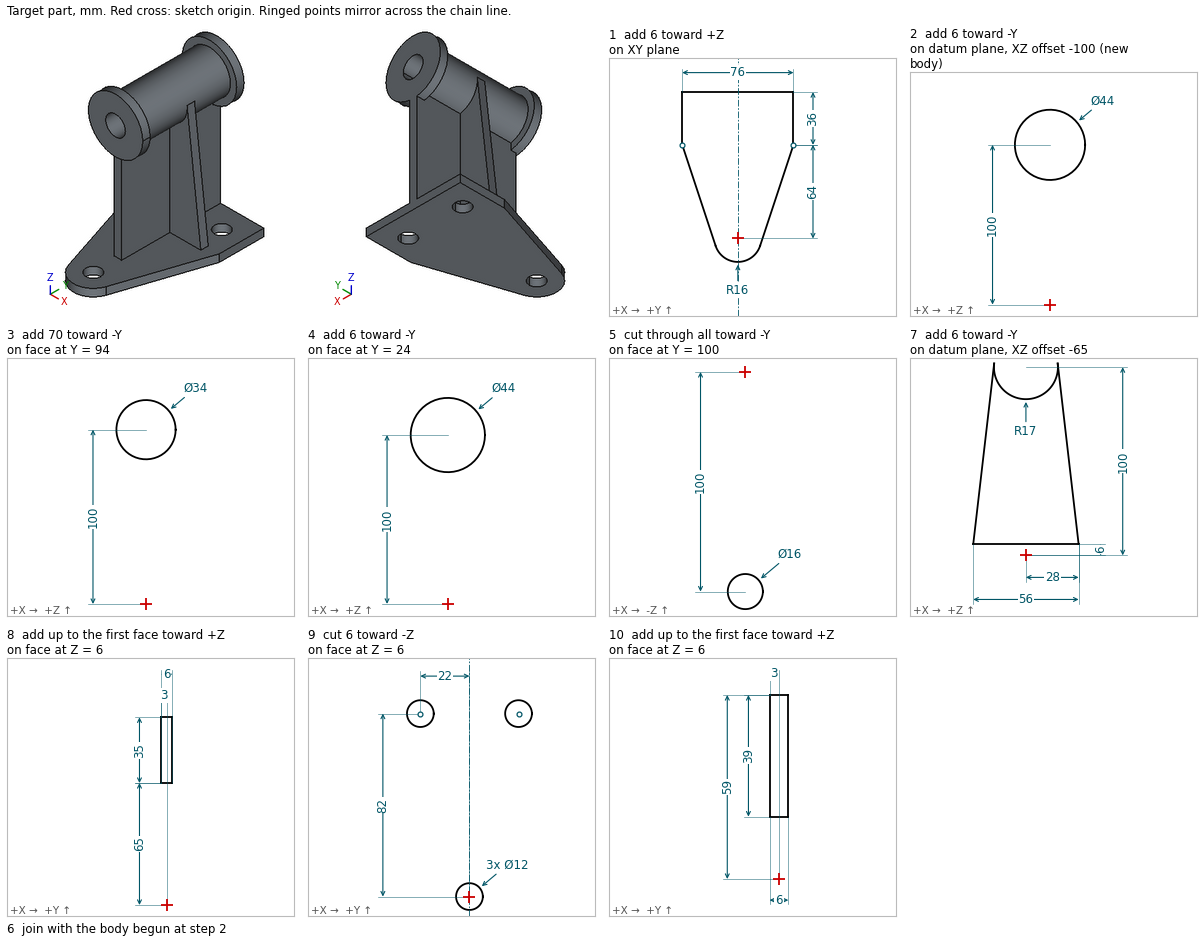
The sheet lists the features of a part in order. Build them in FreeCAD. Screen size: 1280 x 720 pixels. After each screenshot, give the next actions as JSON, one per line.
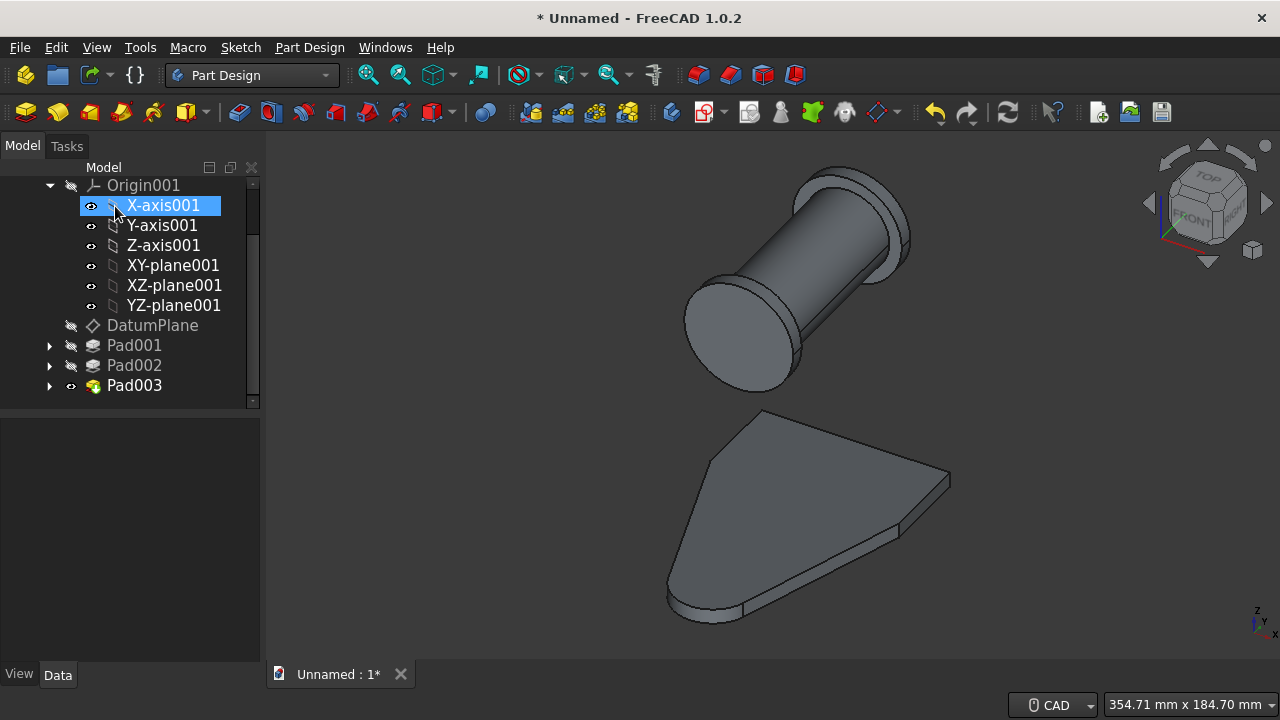
{"action": "key", "text": "4"}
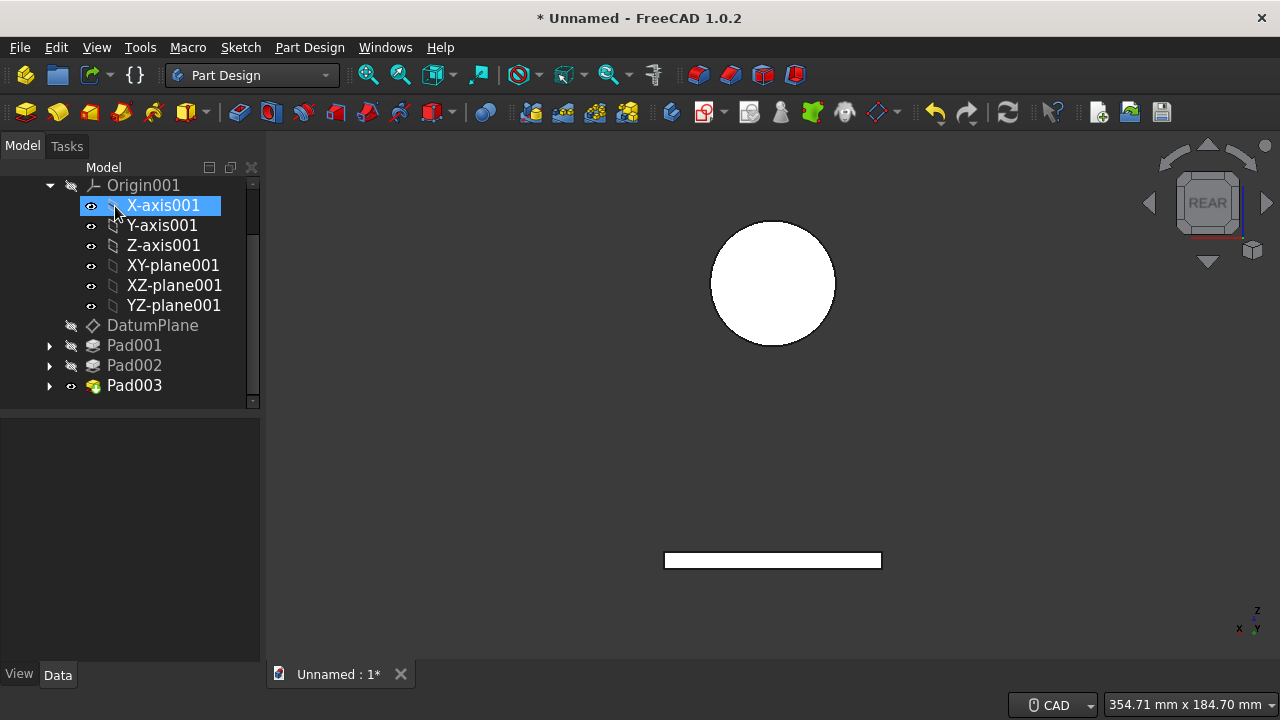
{"action": "left_click", "coordinate": [370, 76]}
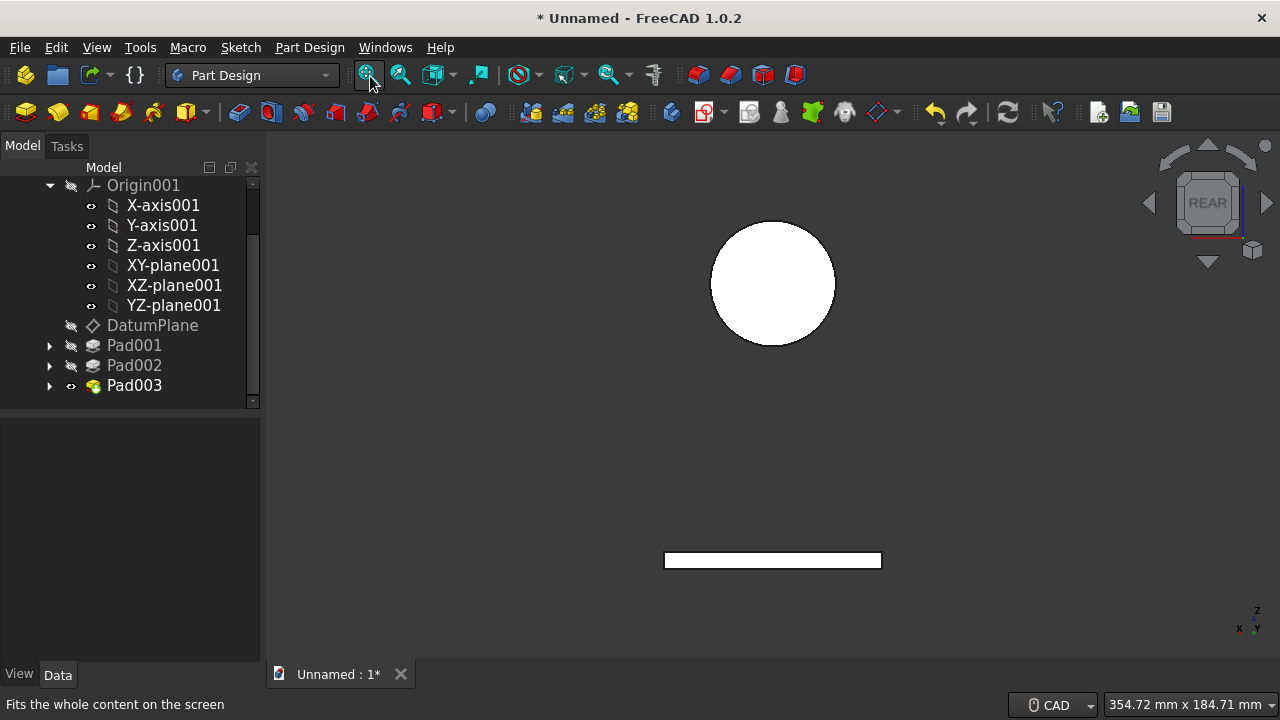
{"action": "left_click", "coordinate": [773, 283]}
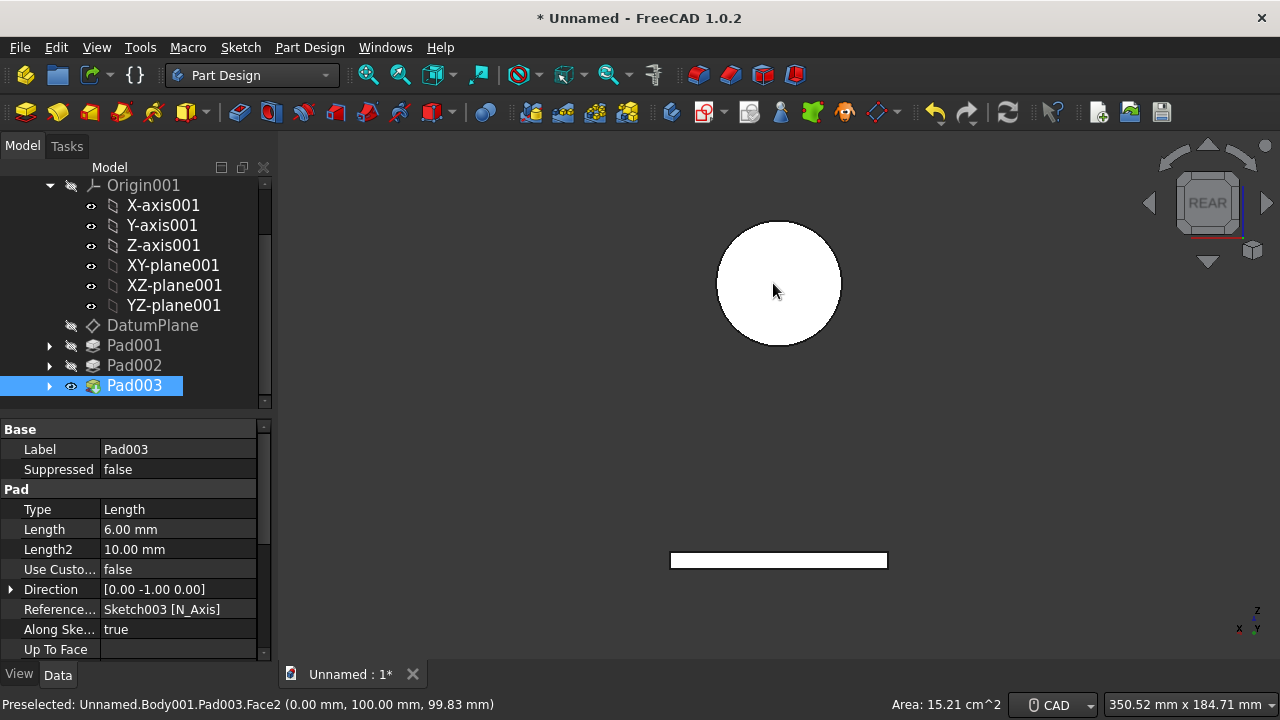
{"action": "left_click", "coordinate": [704, 112]}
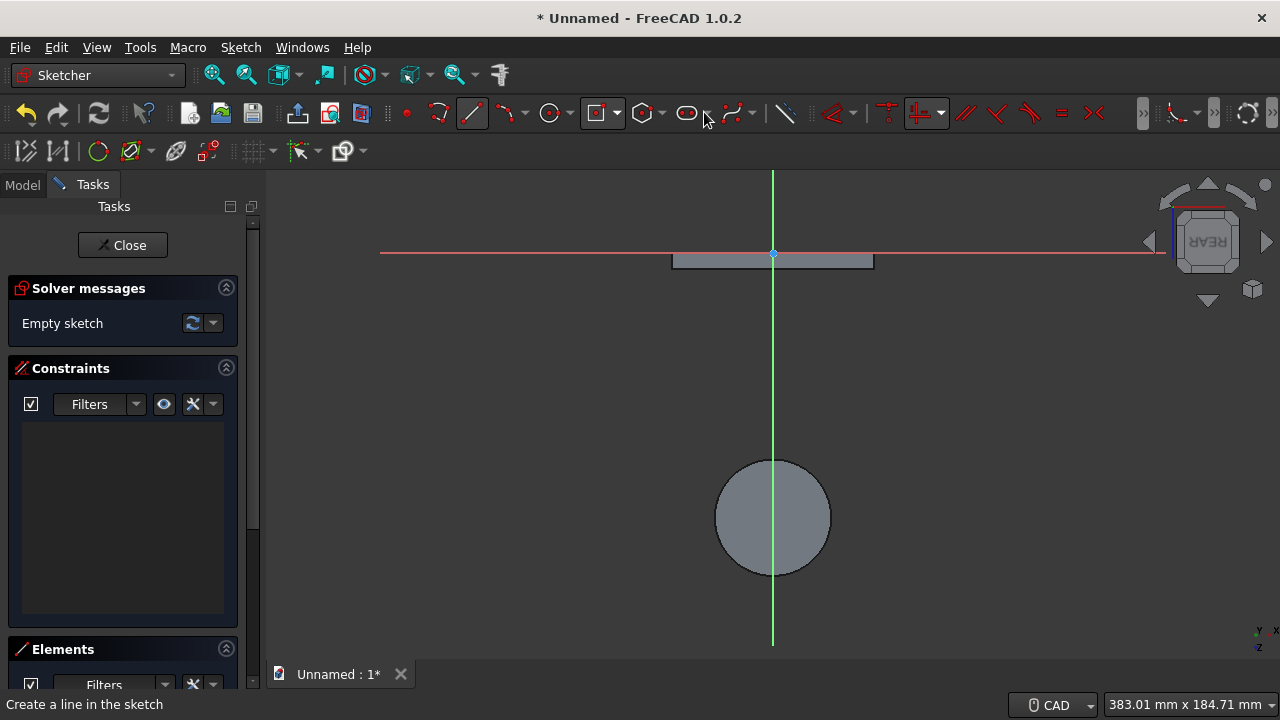
{"action": "scroll", "coordinate": [784, 534], "scroll_direction": "up", "scroll_amount": 10}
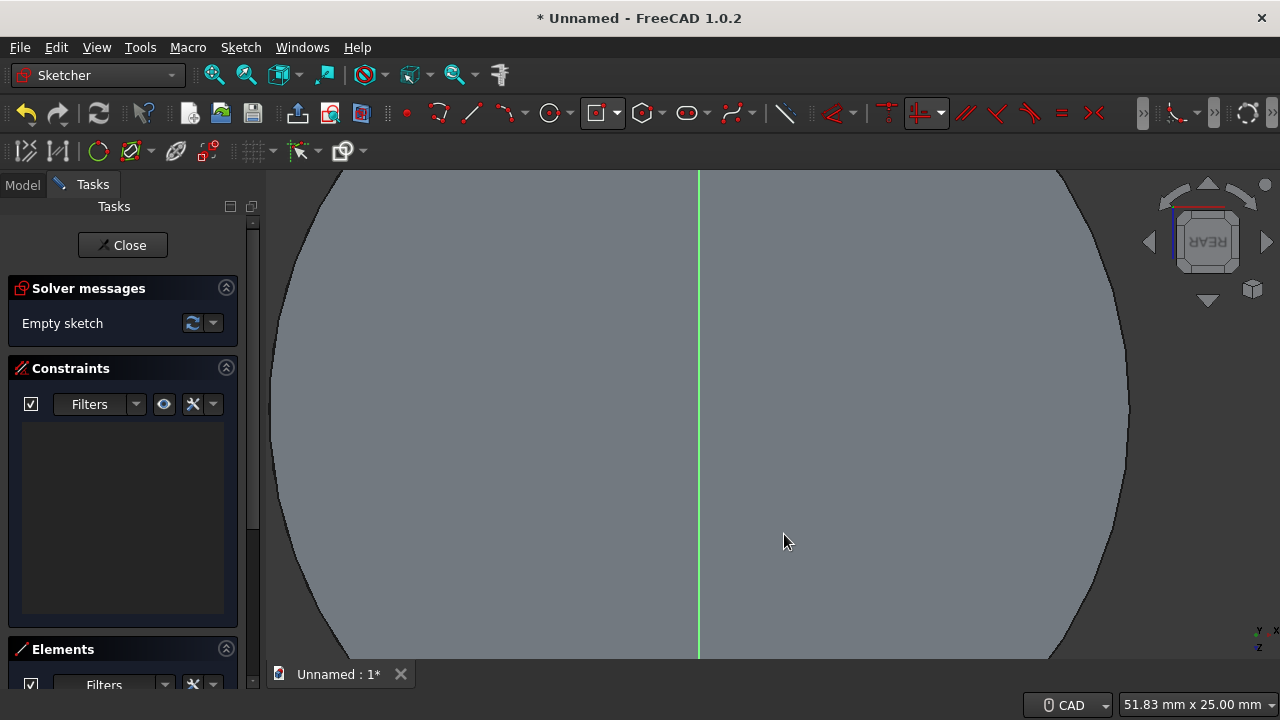
{"action": "key", "text": "g c"}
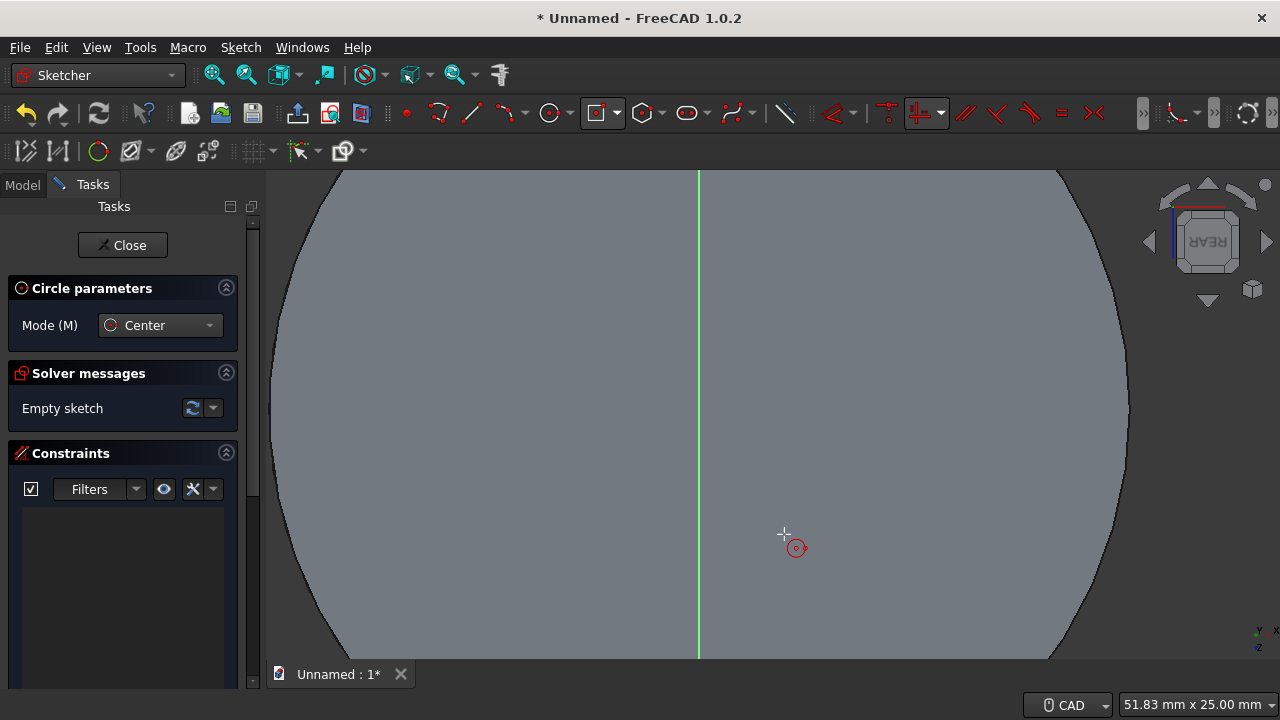
{"action": "left_click", "coordinate": [699, 409]}
{"action": "left_click", "coordinate": [810, 299]}
{"action": "key", "text": "Escape"}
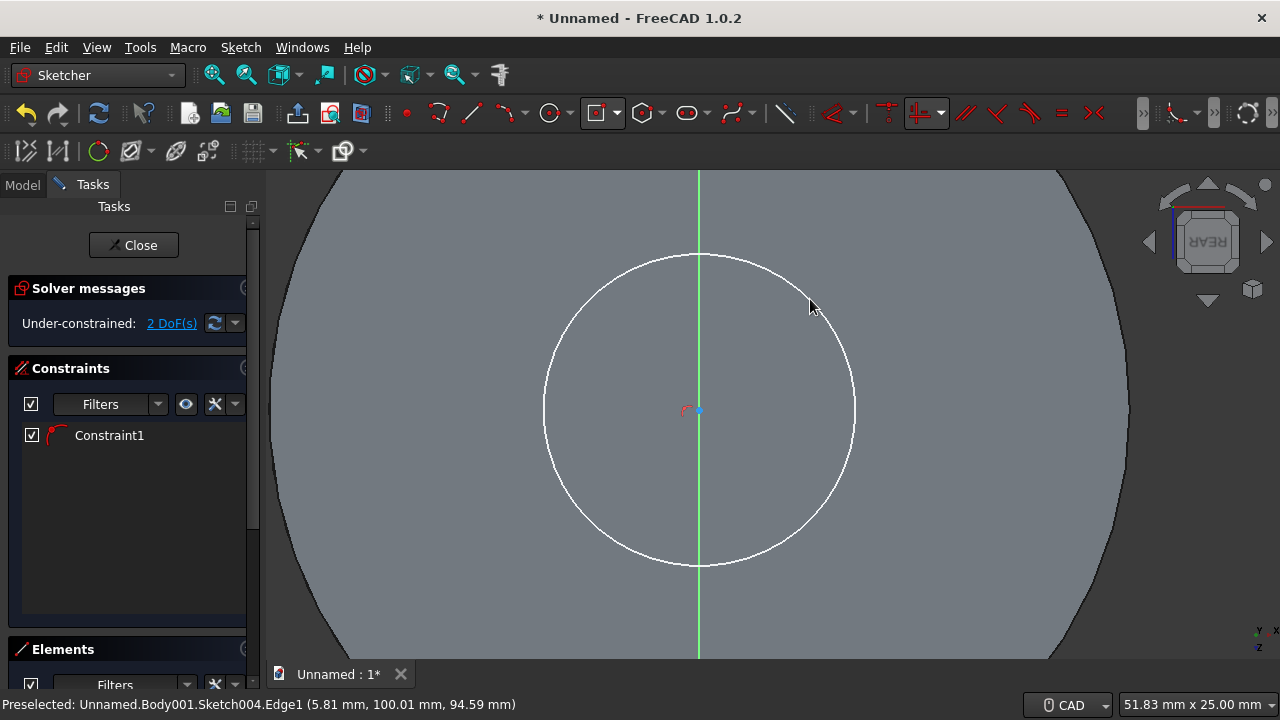
{"action": "key", "text": "d"}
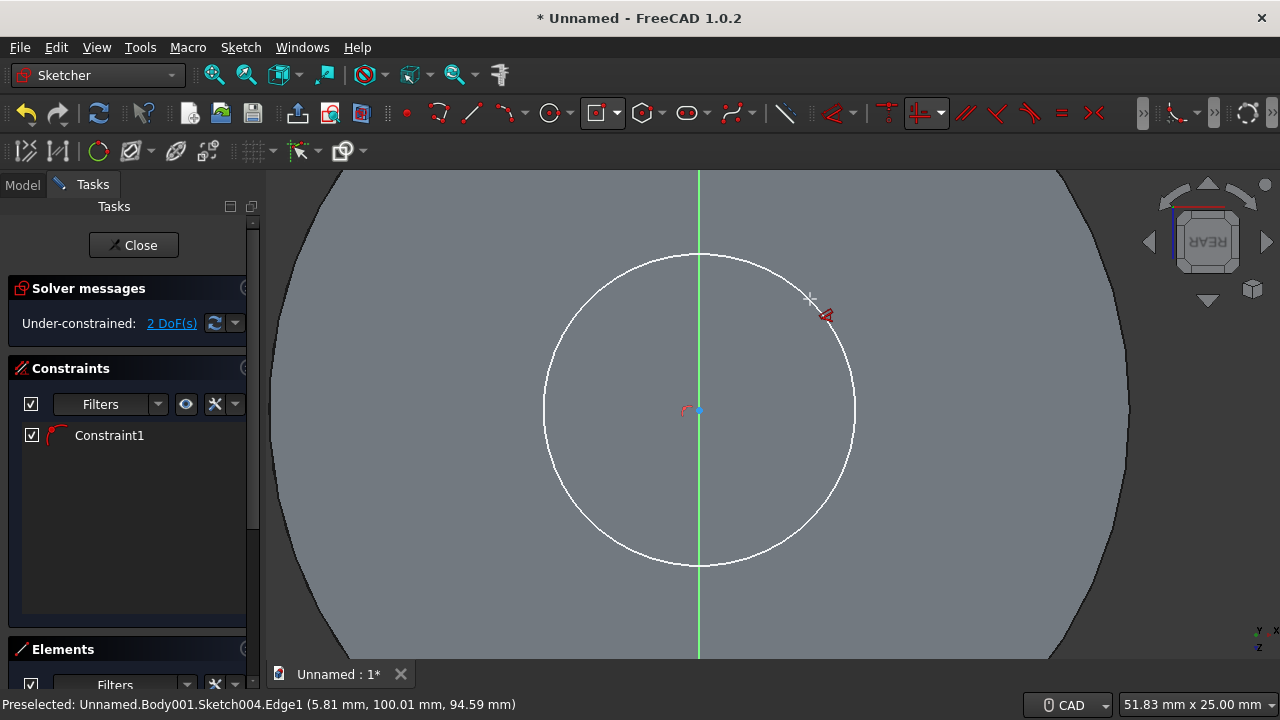
{"action": "left_click", "coordinate": [809, 299]}
{"action": "left_click", "coordinate": [831, 276]}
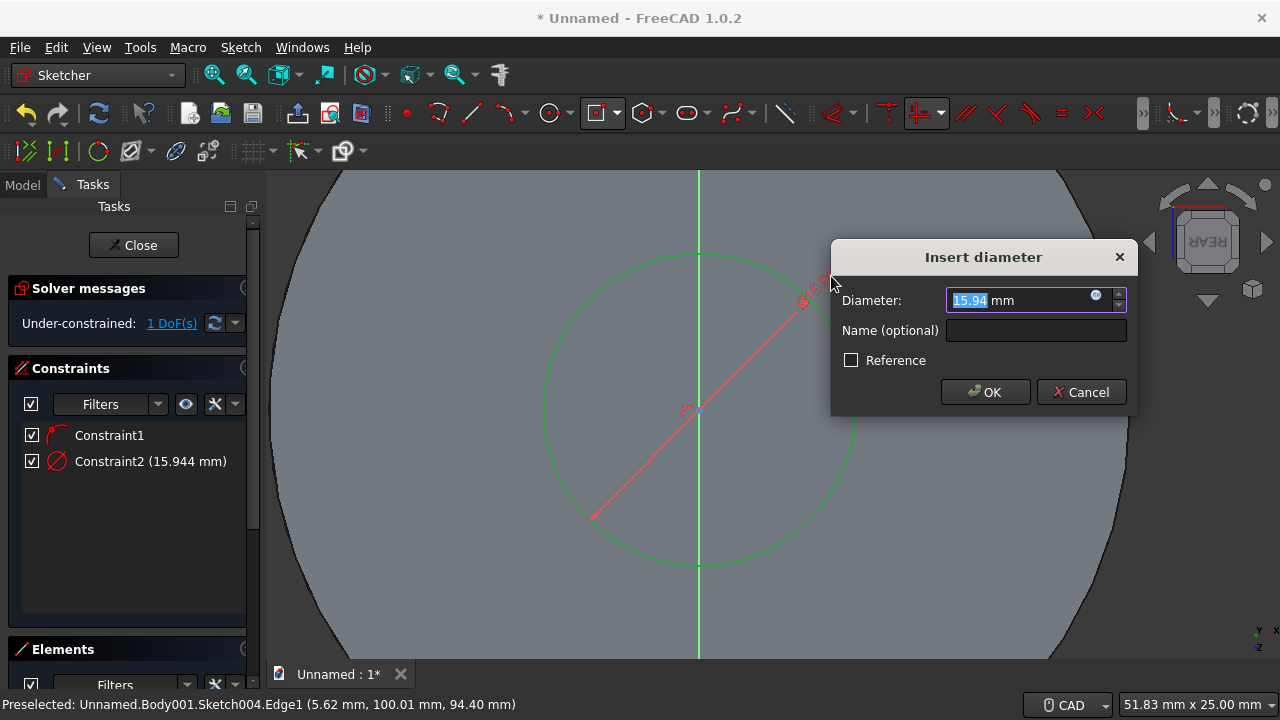
{"action": "type", "text": "16"}
{"action": "key", "text": "Return"}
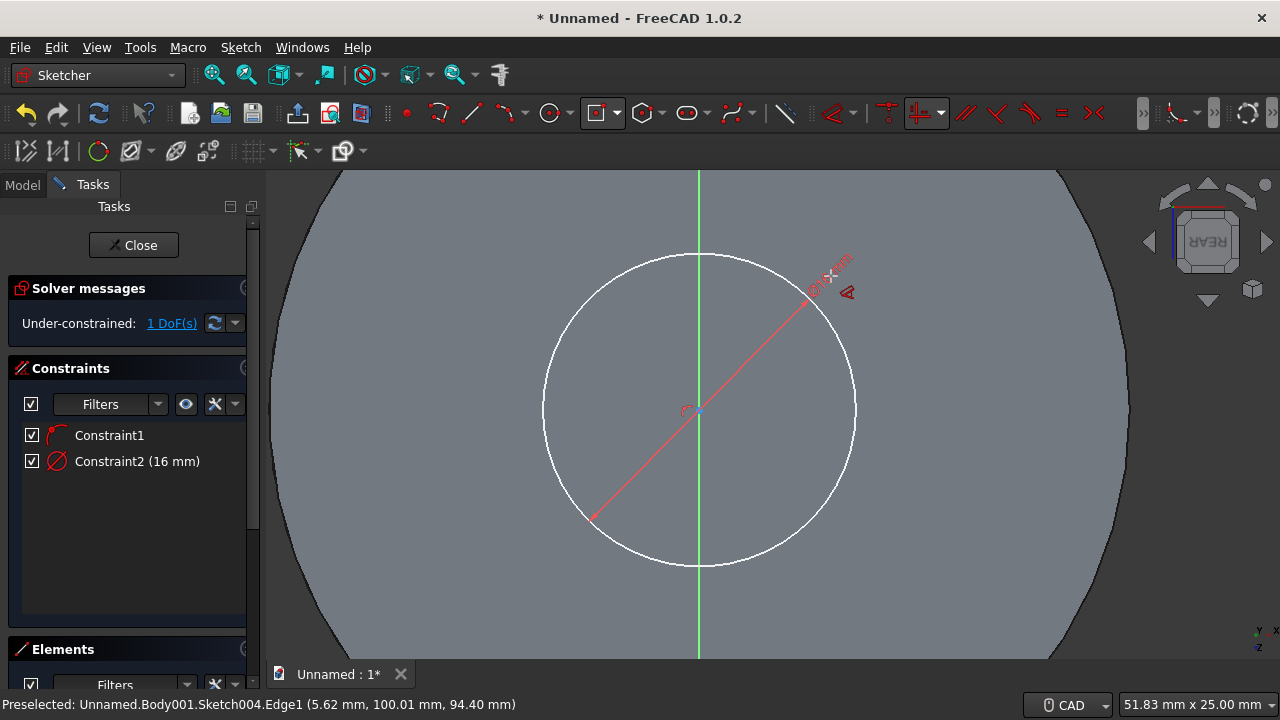
{"action": "left_click", "coordinate": [699, 410]}
{"action": "left_click", "coordinate": [733, 304]}